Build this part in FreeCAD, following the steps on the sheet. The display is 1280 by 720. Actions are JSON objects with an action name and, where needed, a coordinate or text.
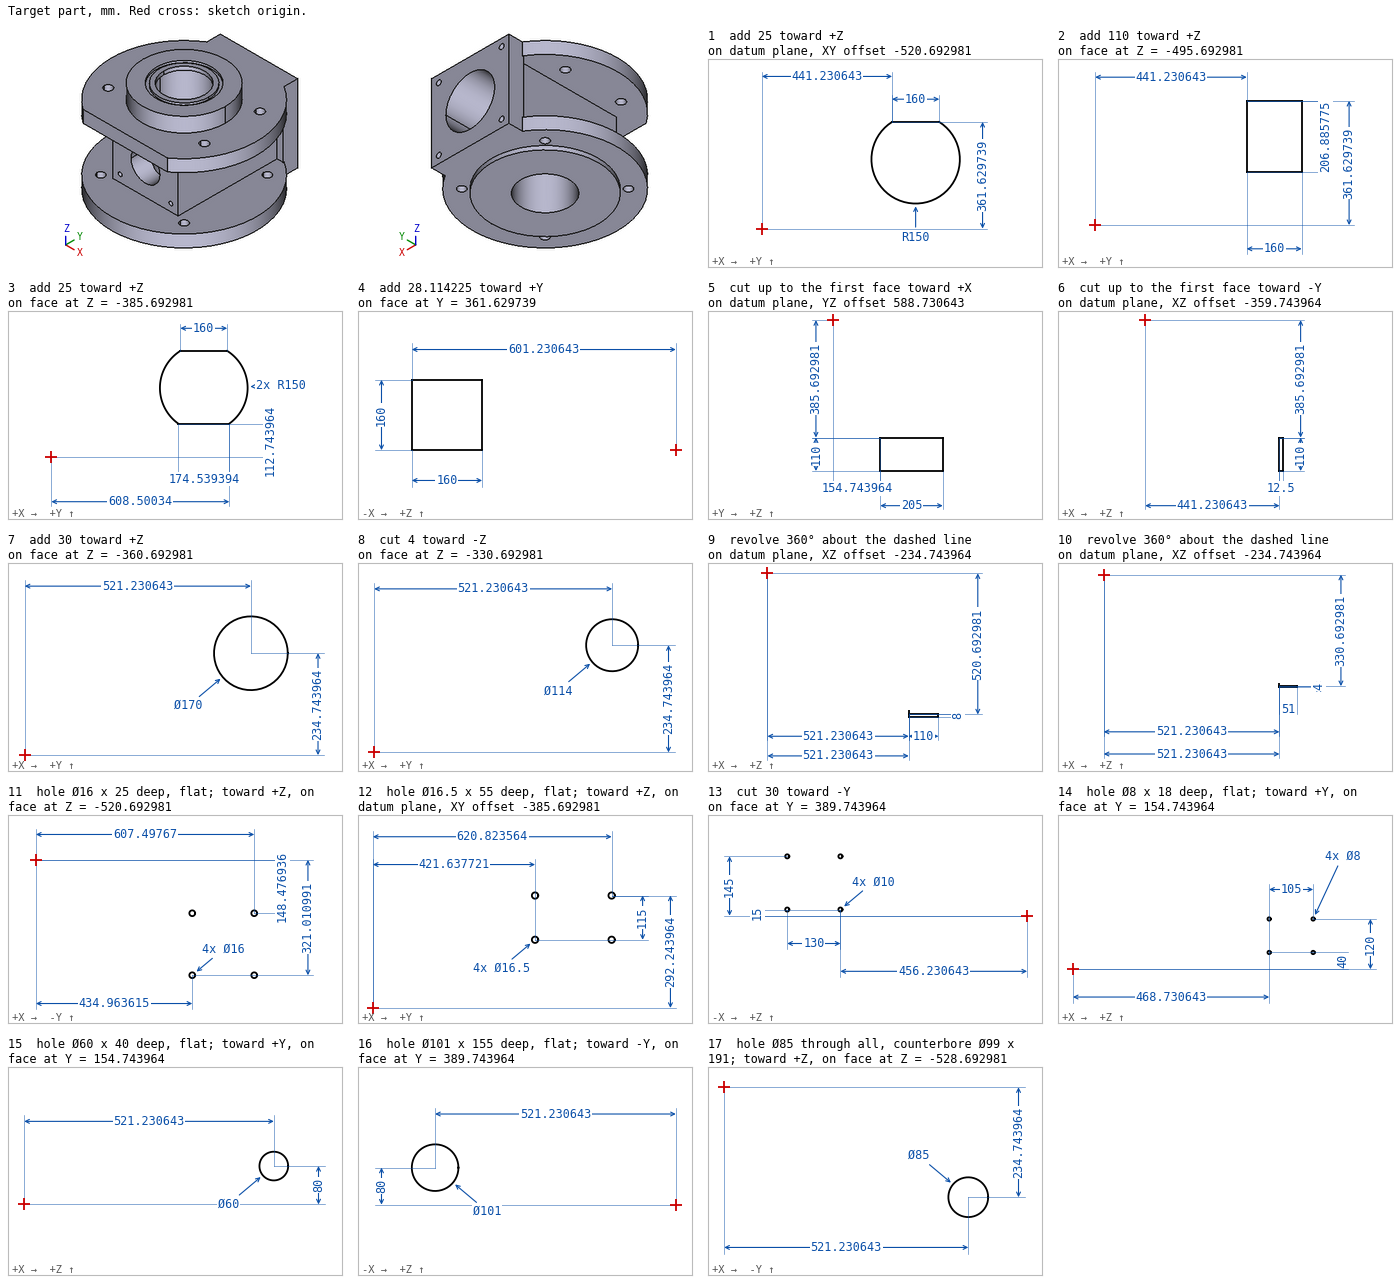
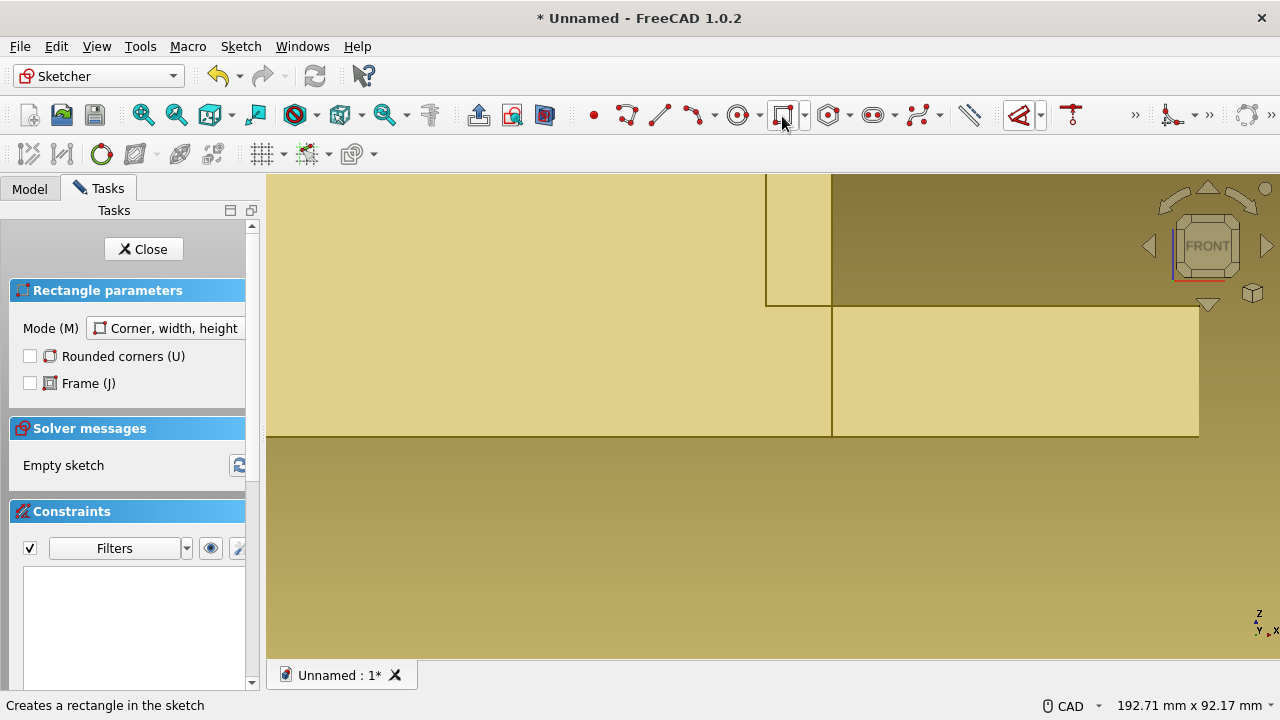
{"action": "left_click", "coordinate": [411, 437]}
{"action": "left_click", "coordinate": [990, 479]}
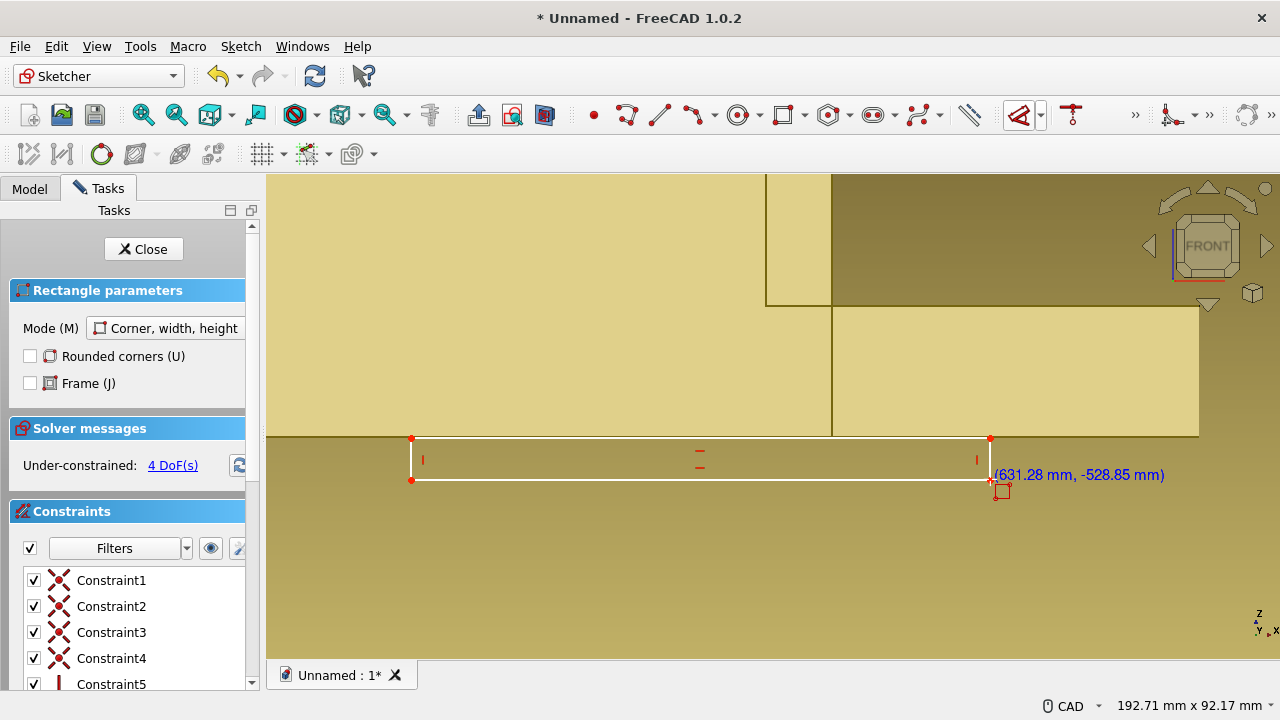
{"action": "left_click", "coordinate": [660, 116]}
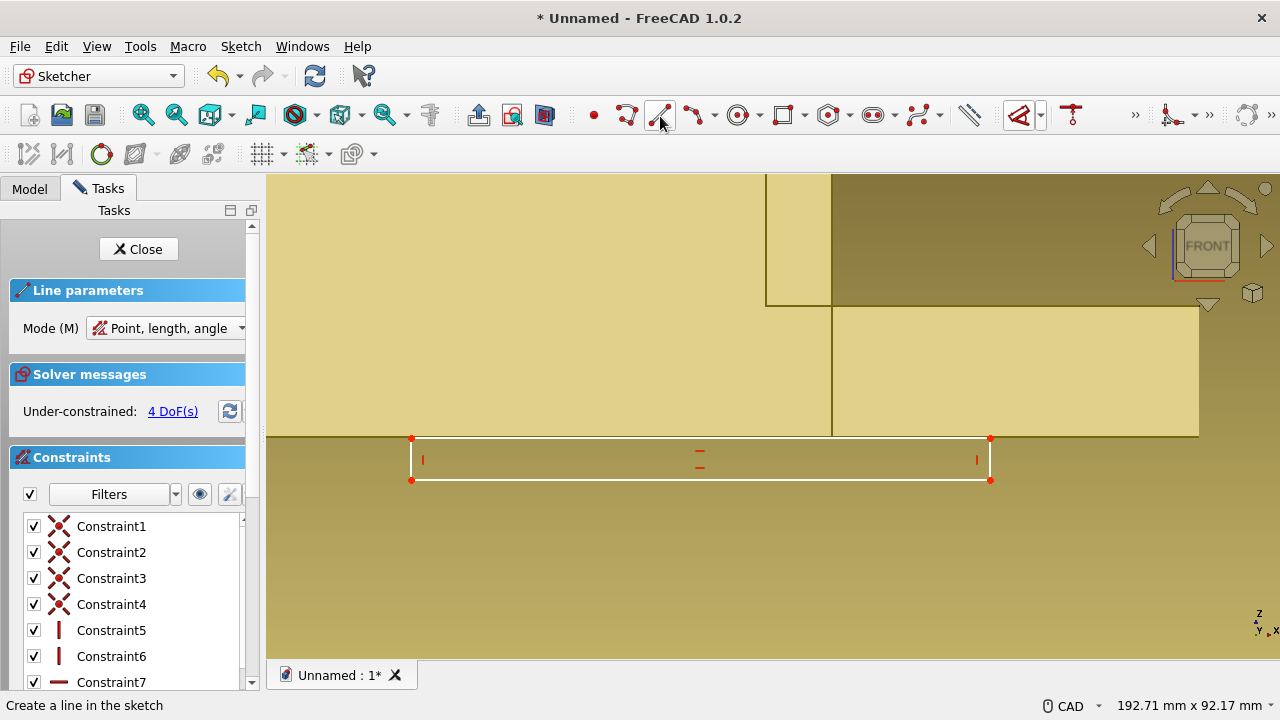
{"action": "left_click", "coordinate": [411, 414]}
{"action": "left_click", "coordinate": [411, 344]}
{"action": "key", "text": "Escape"}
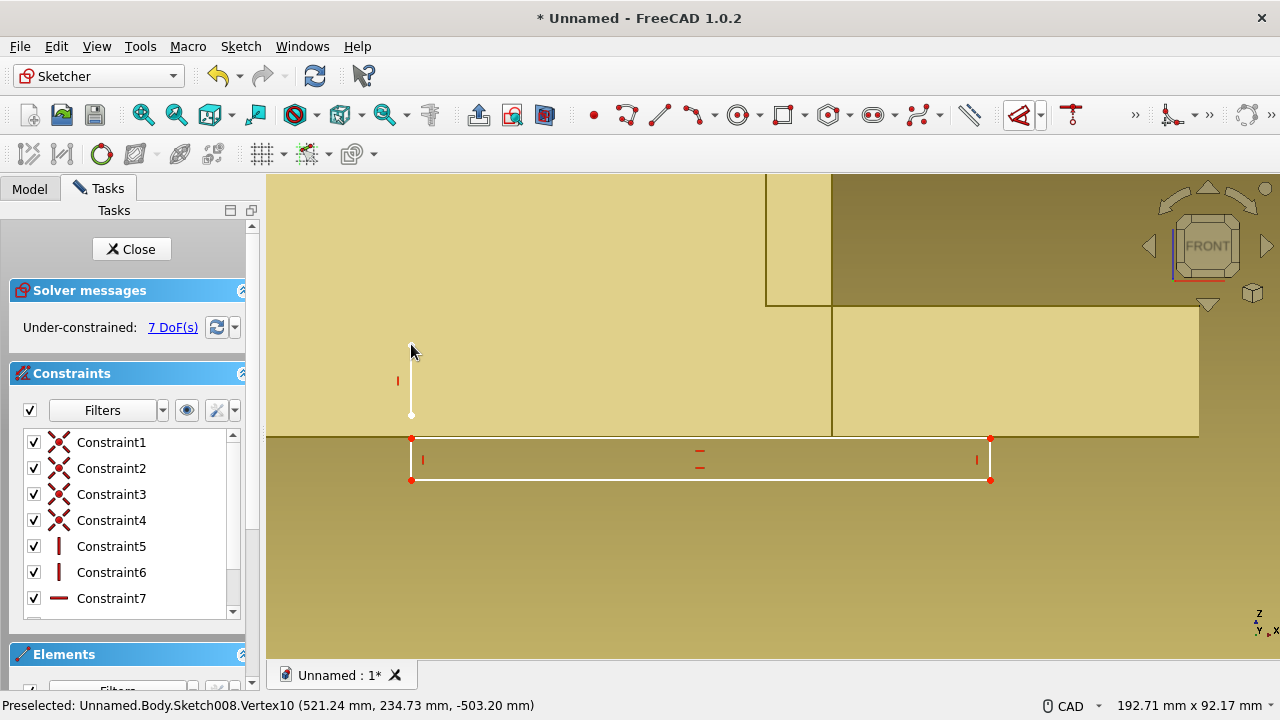
{"action": "left_click", "coordinate": [411, 394]}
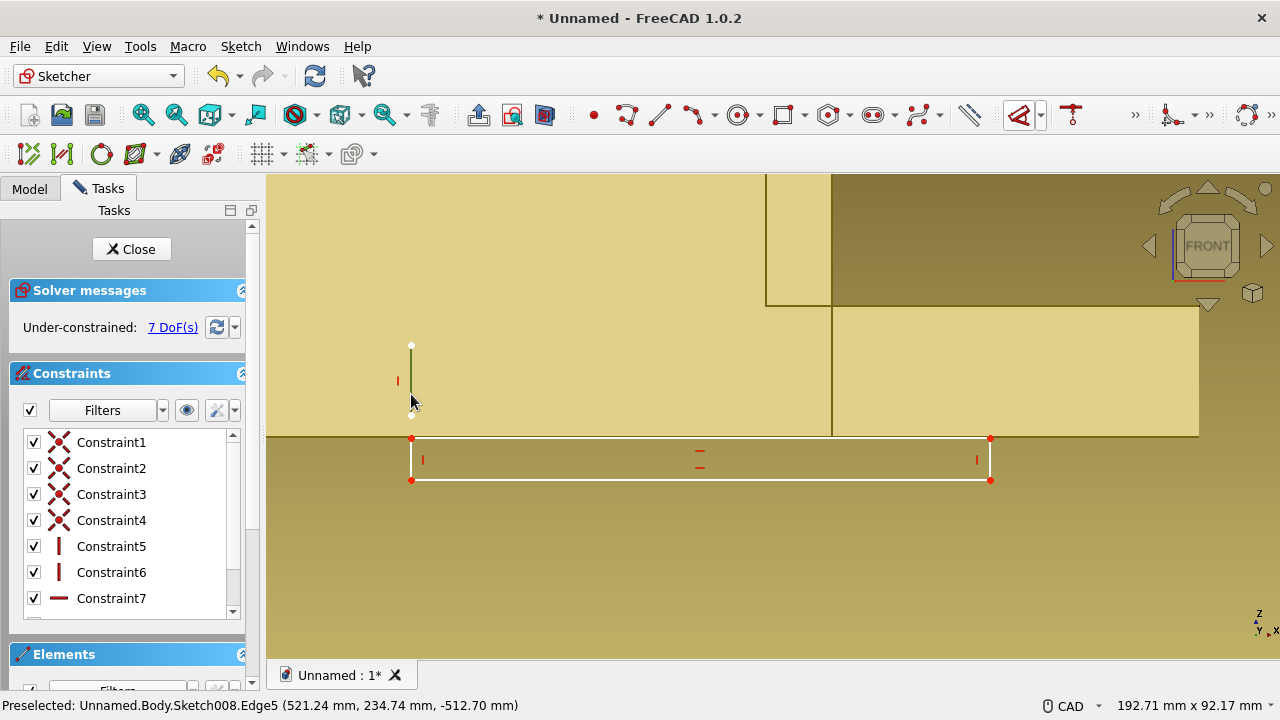
{"action": "left_click", "coordinate": [970, 116]}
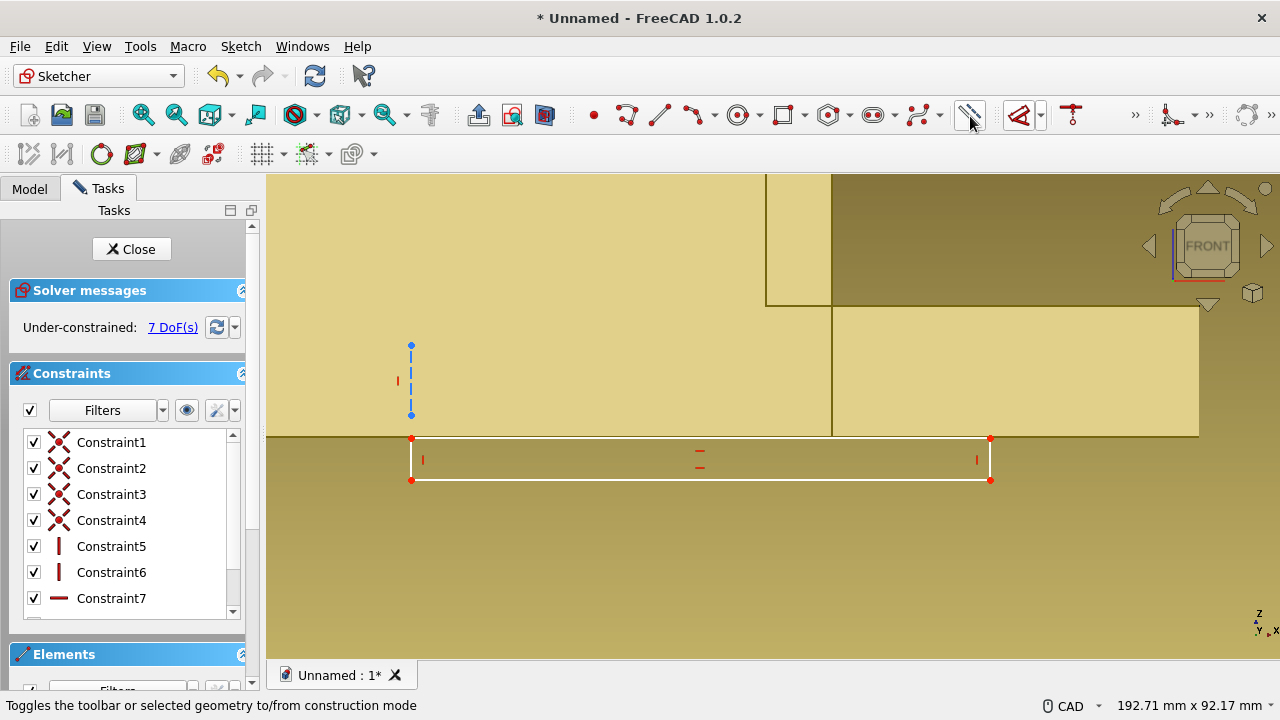
{"action": "left_click", "coordinate": [411, 451]}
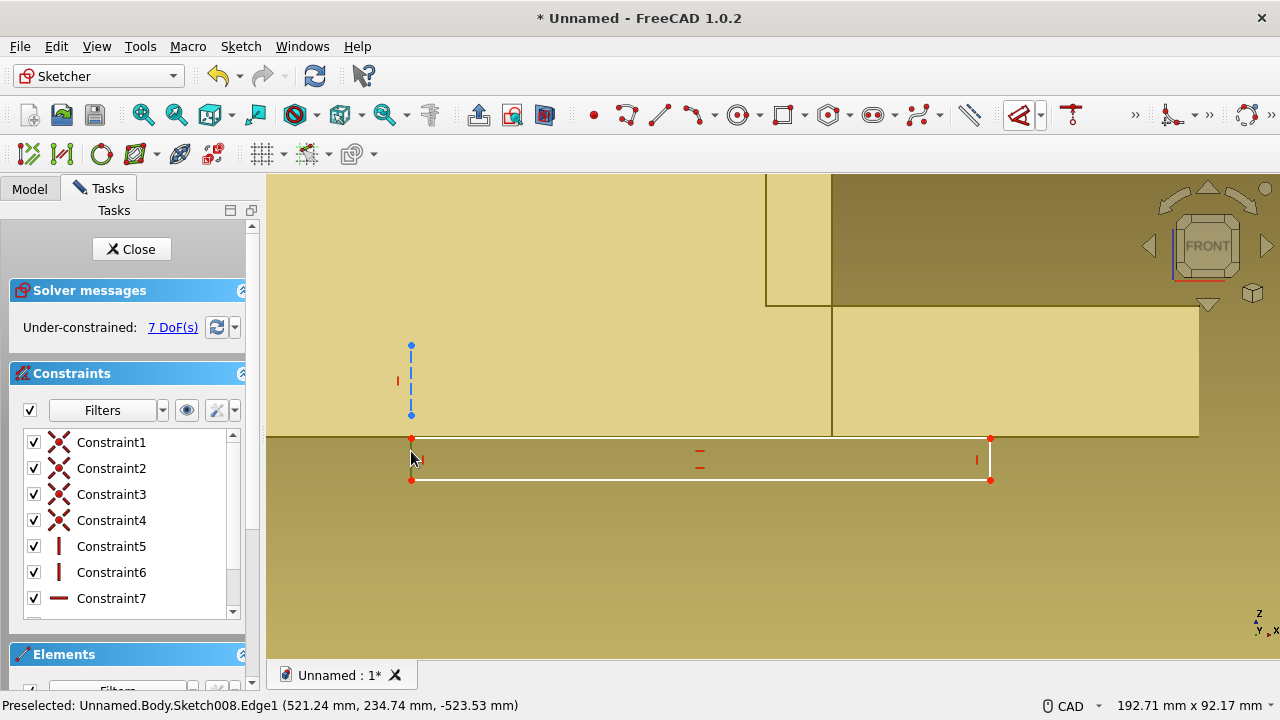
{"action": "left_click", "coordinate": [1040, 116]}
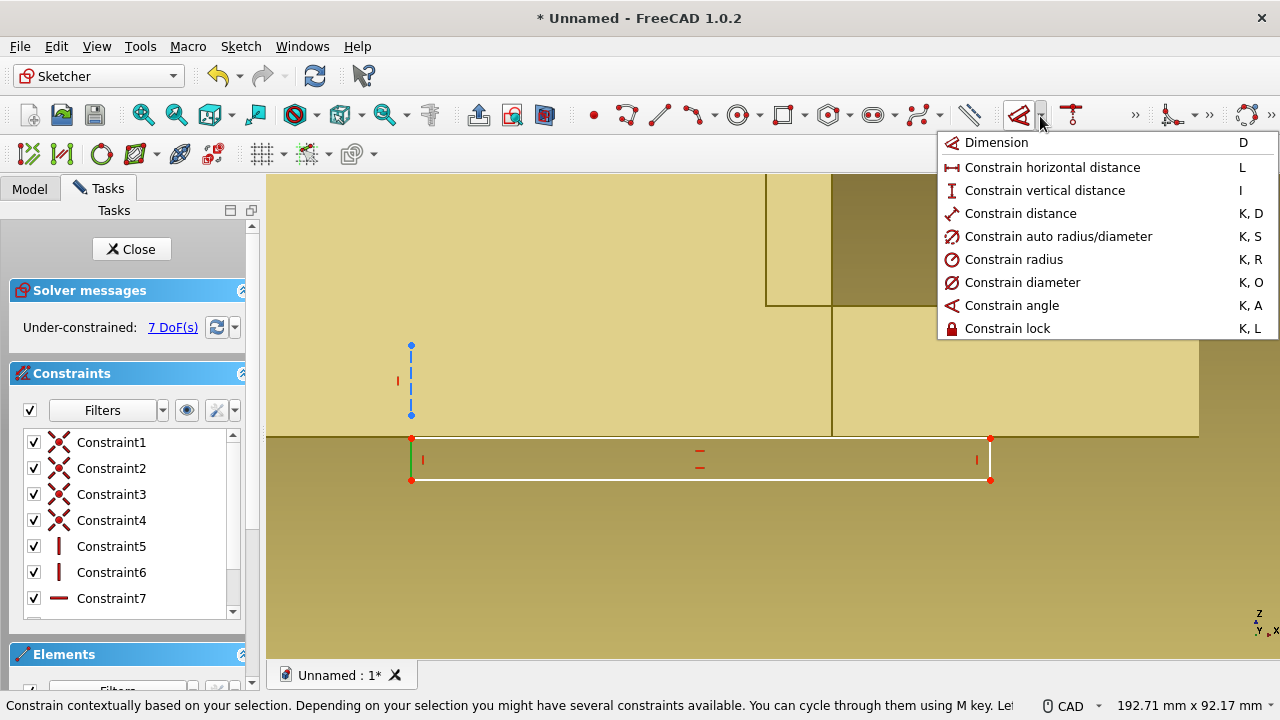
{"action": "left_click", "coordinate": [1108, 190]}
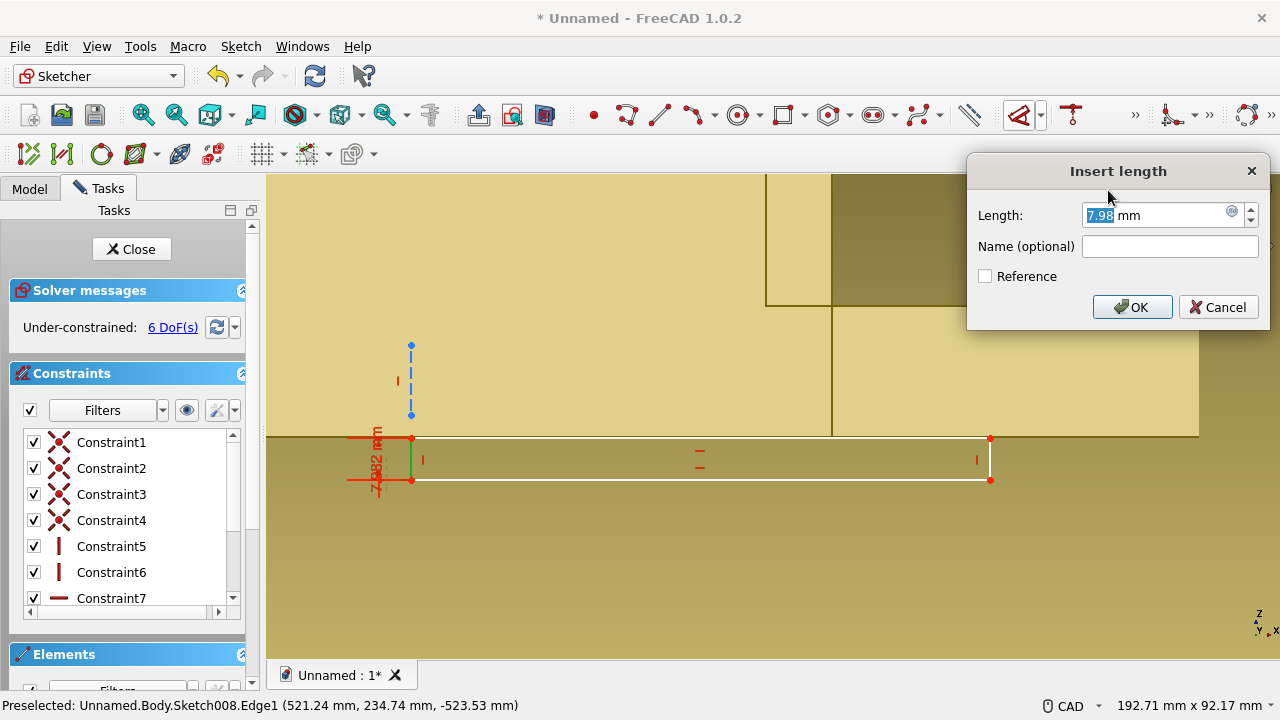
{"action": "type", "text": "8"}
{"action": "key", "text": "Return"}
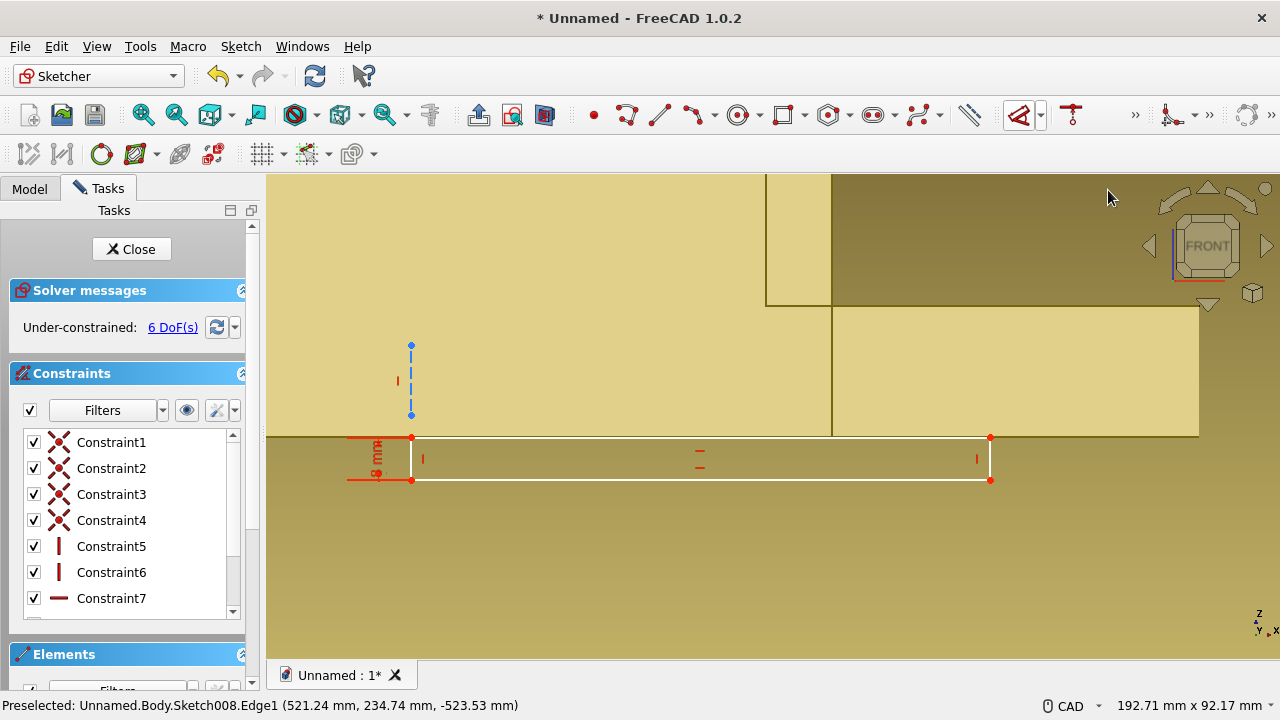
{"action": "left_click", "coordinate": [585, 480]}